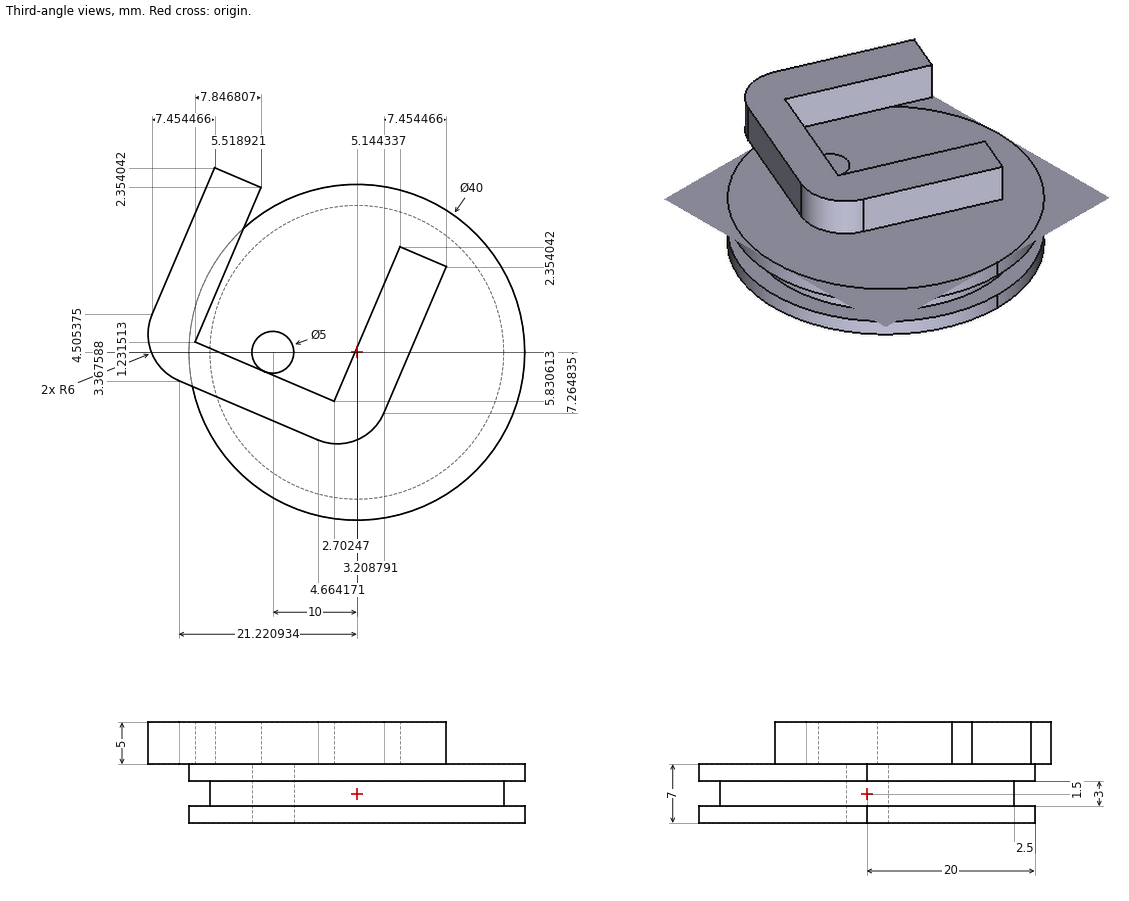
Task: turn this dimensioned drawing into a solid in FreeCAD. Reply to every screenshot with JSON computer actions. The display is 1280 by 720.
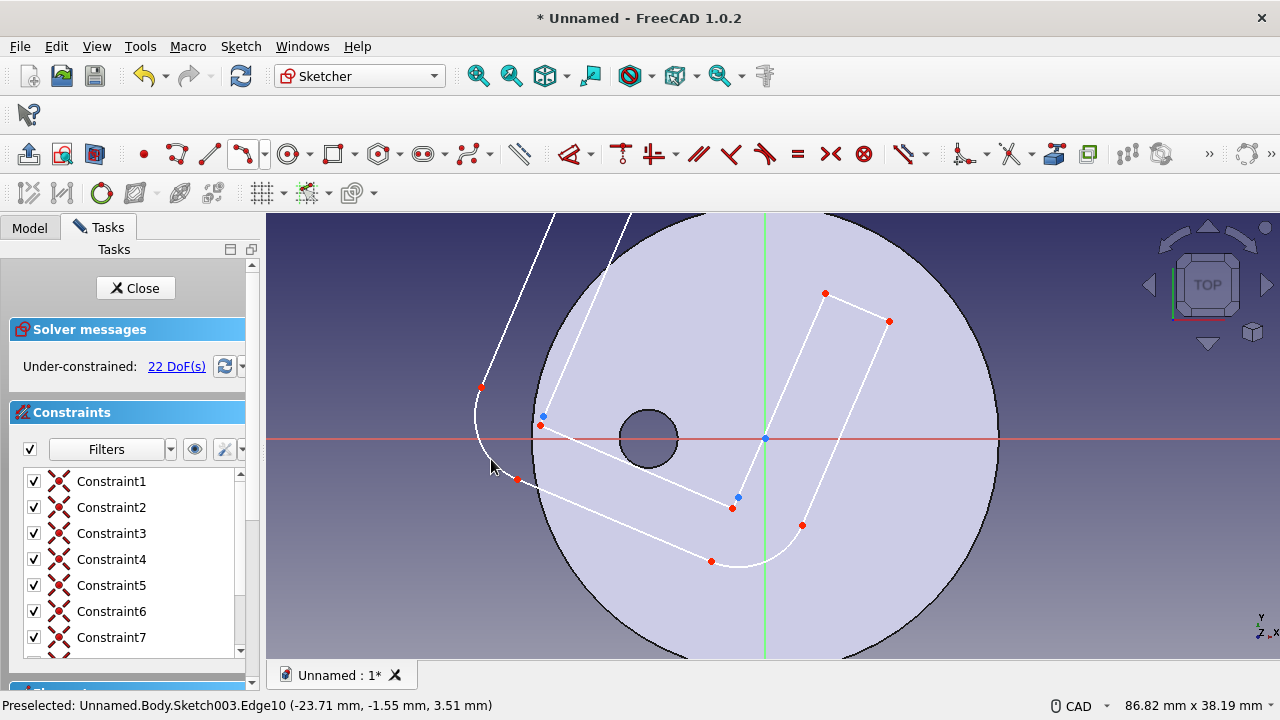
{"action": "left_click", "coordinate": [576, 504]}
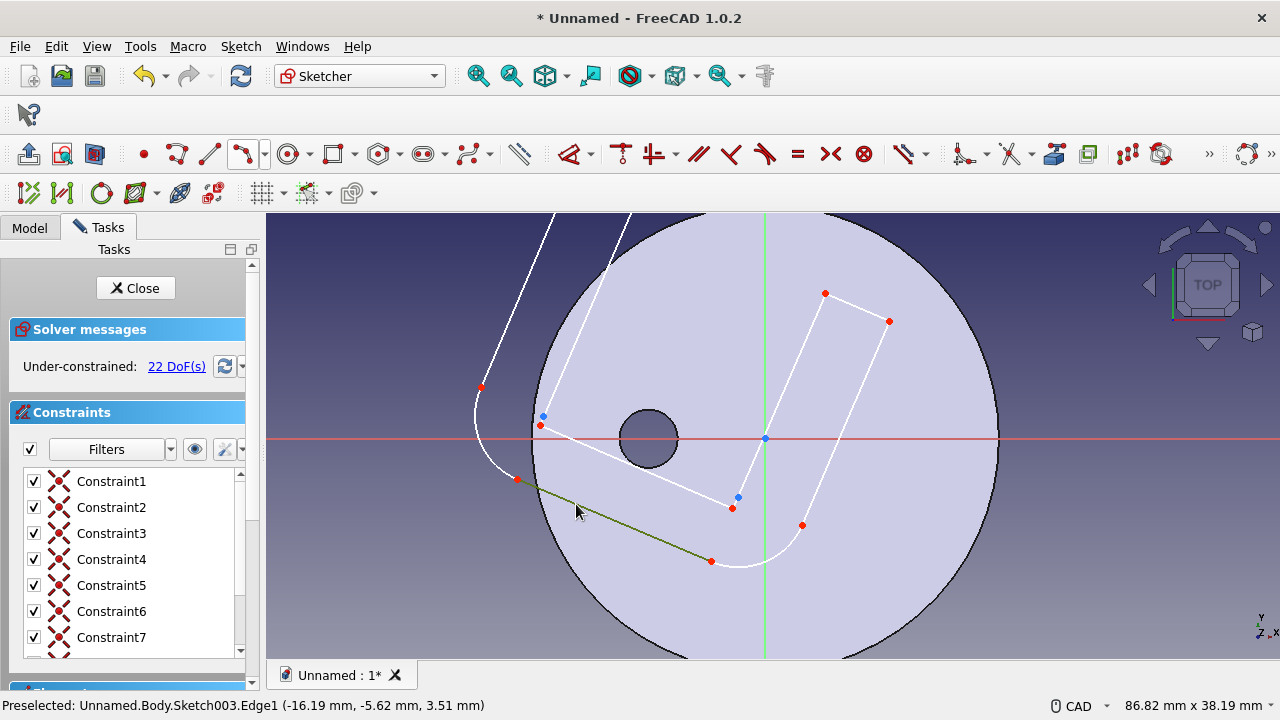
{"action": "left_click", "coordinate": [743, 567]}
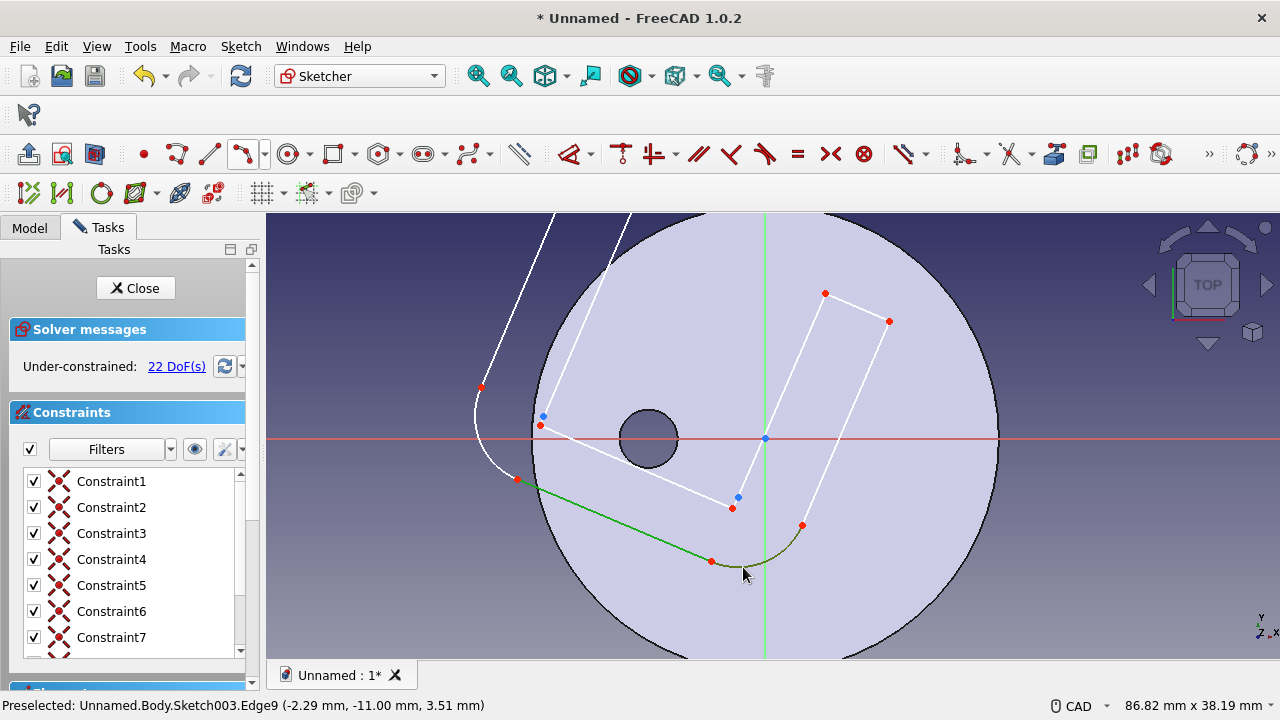
{"action": "left_click", "coordinate": [765, 154]}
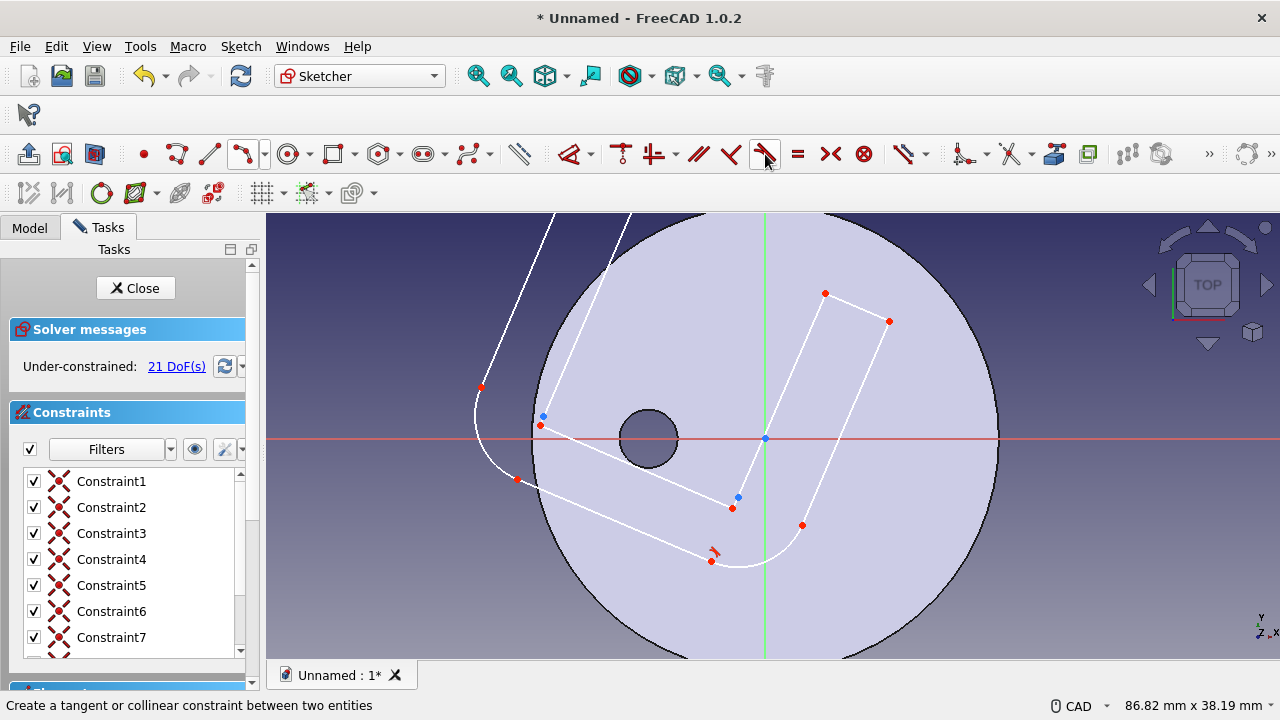
{"action": "left_click", "coordinate": [576, 504]}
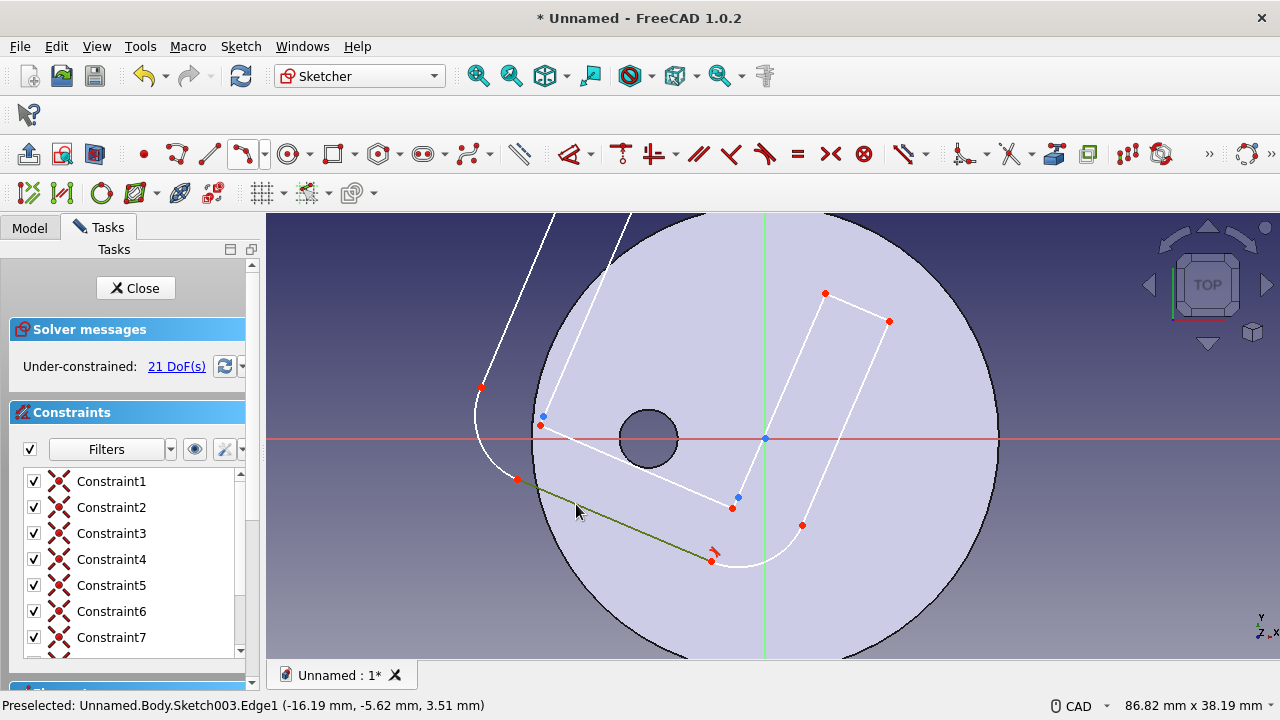
{"action": "left_click", "coordinate": [475, 420]}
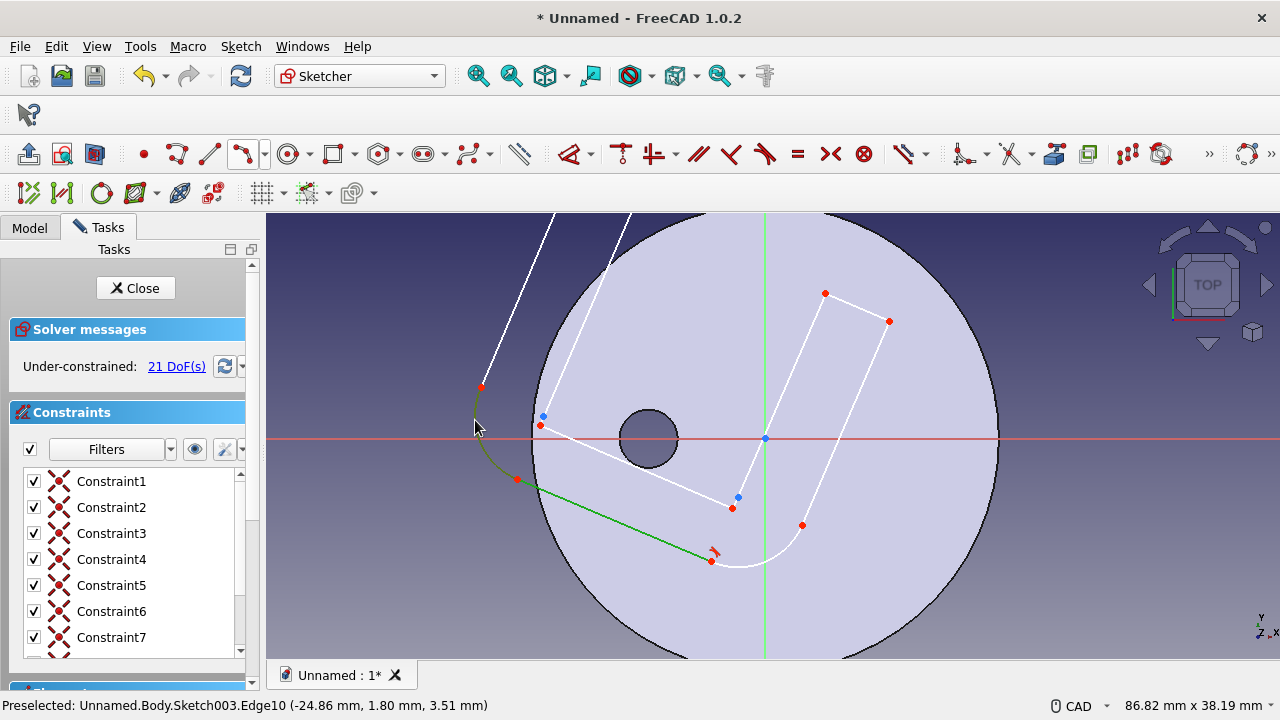
{"action": "left_click", "coordinate": [765, 154]}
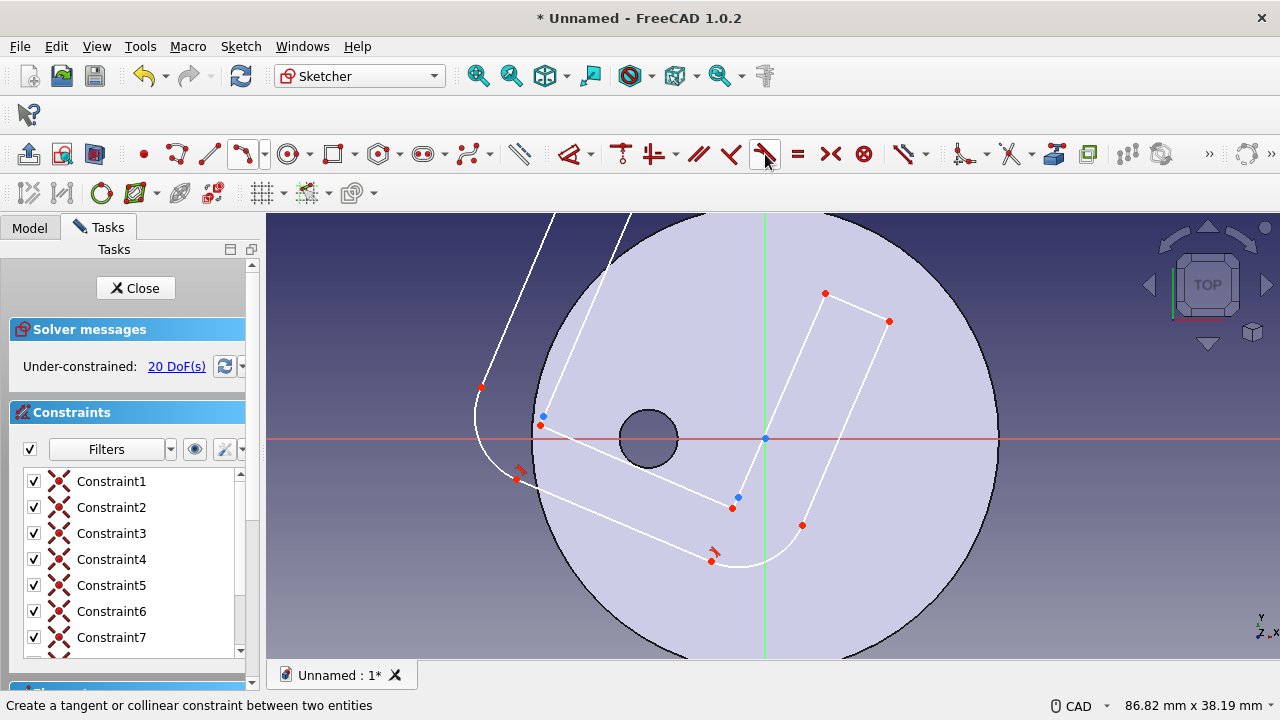
{"action": "left_click", "coordinate": [828, 464]}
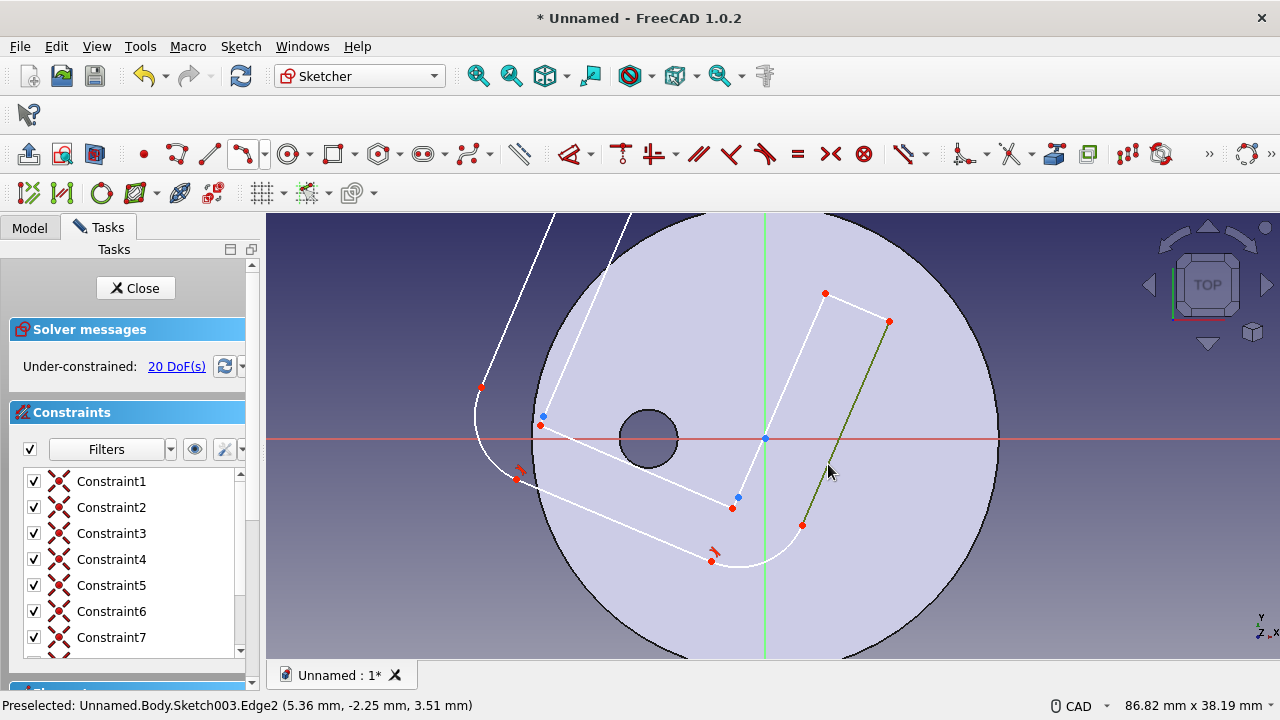
{"action": "left_click", "coordinate": [743, 567]}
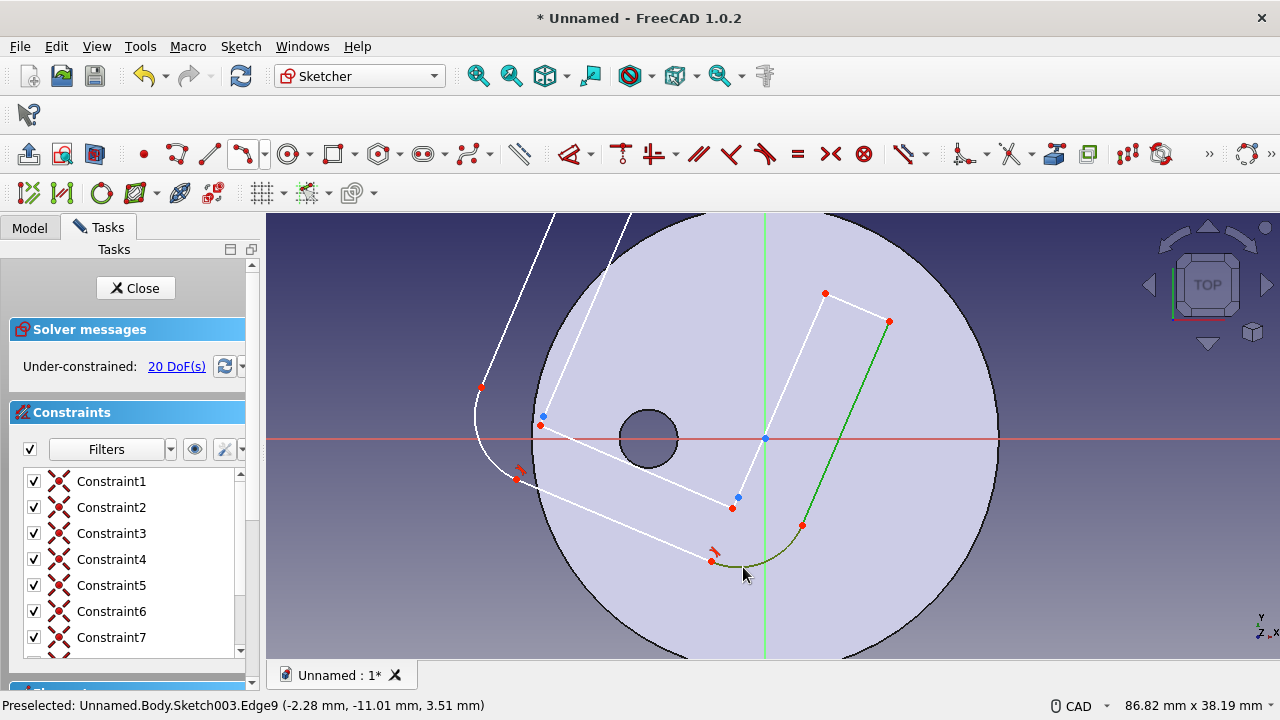
{"action": "left_click", "coordinate": [765, 154]}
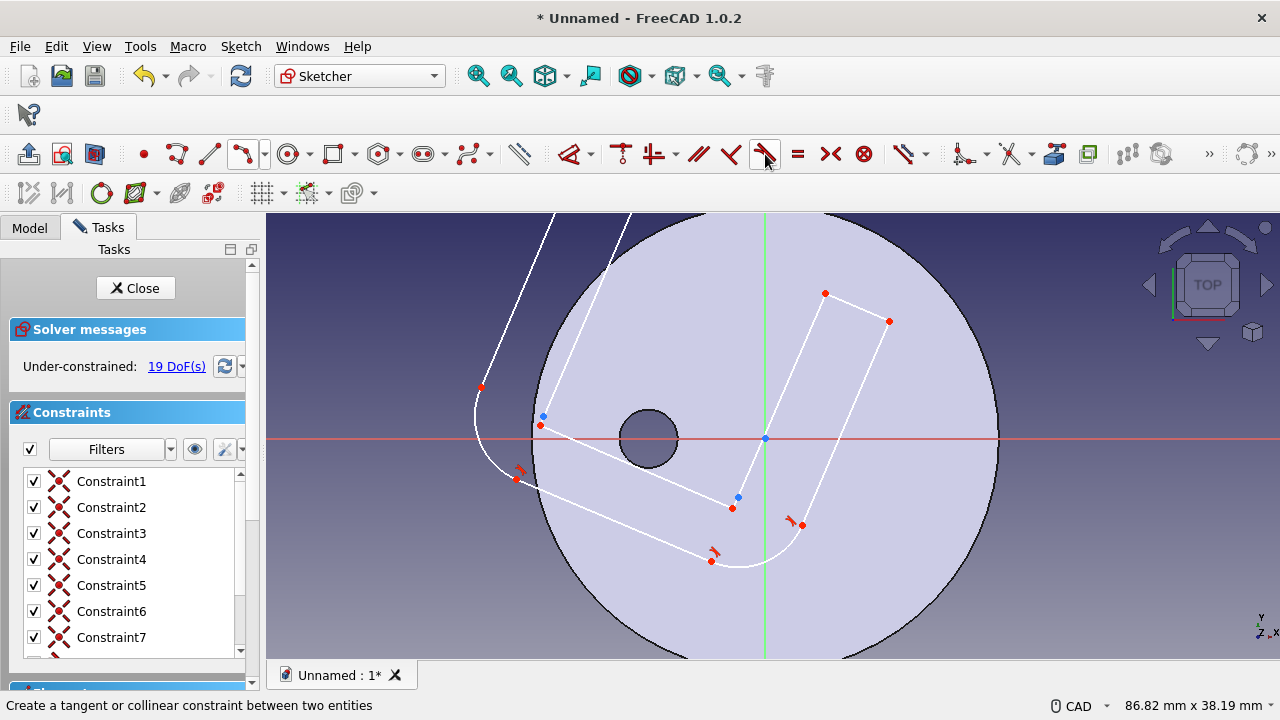
{"action": "left_click", "coordinate": [542, 245]}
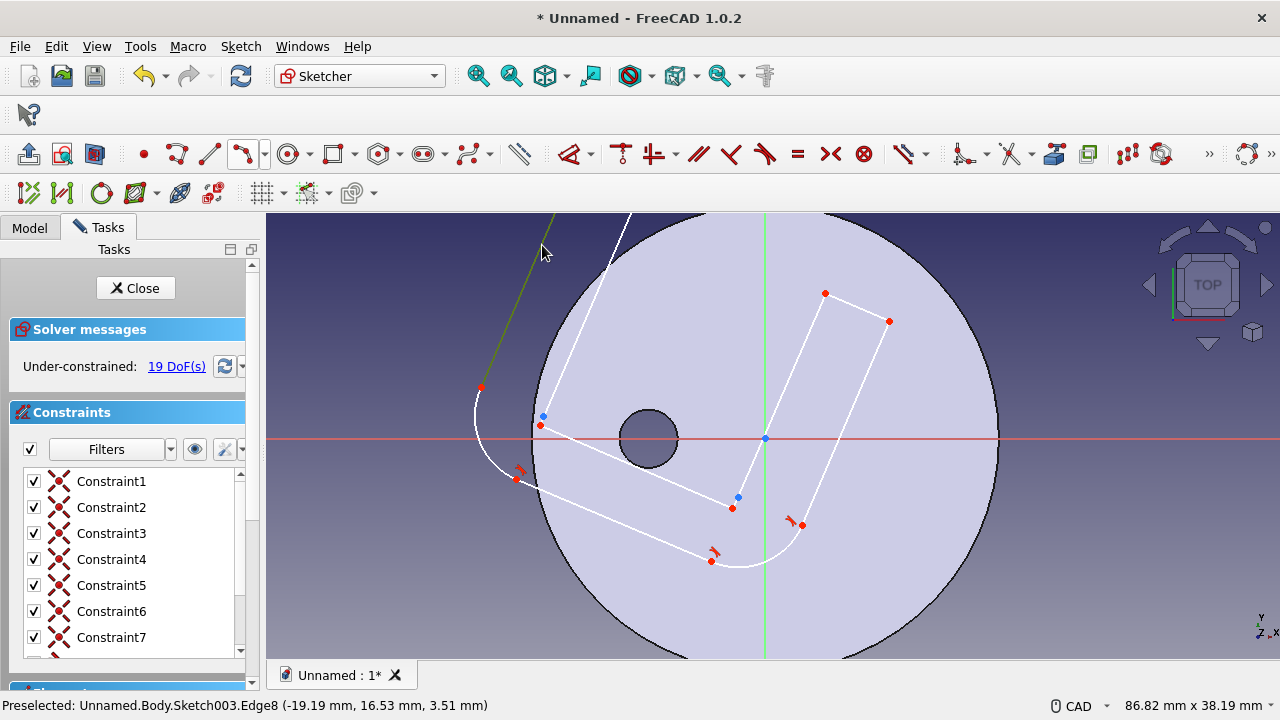
{"action": "left_click", "coordinate": [475, 420]}